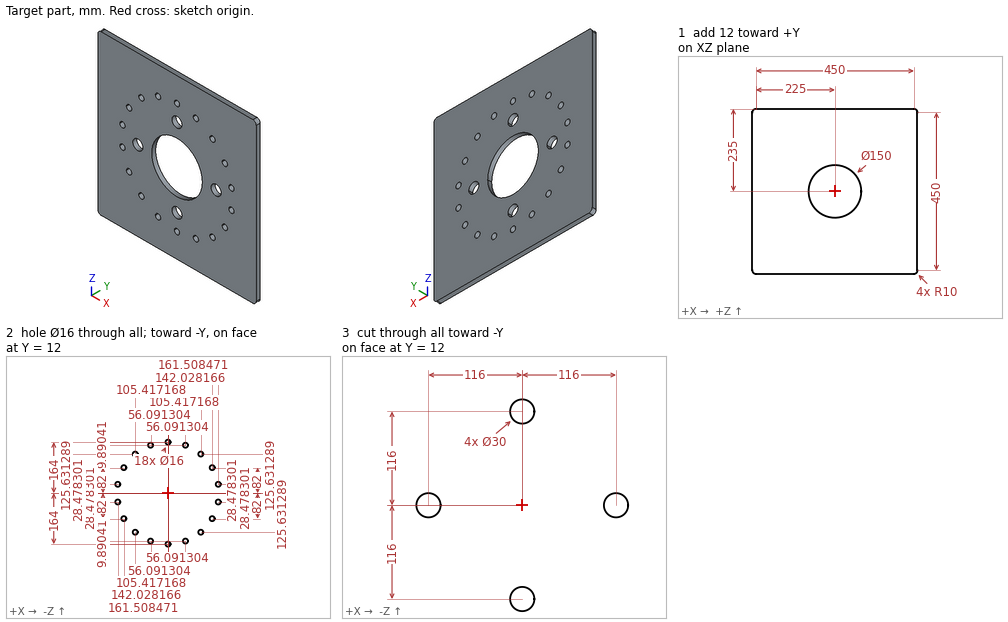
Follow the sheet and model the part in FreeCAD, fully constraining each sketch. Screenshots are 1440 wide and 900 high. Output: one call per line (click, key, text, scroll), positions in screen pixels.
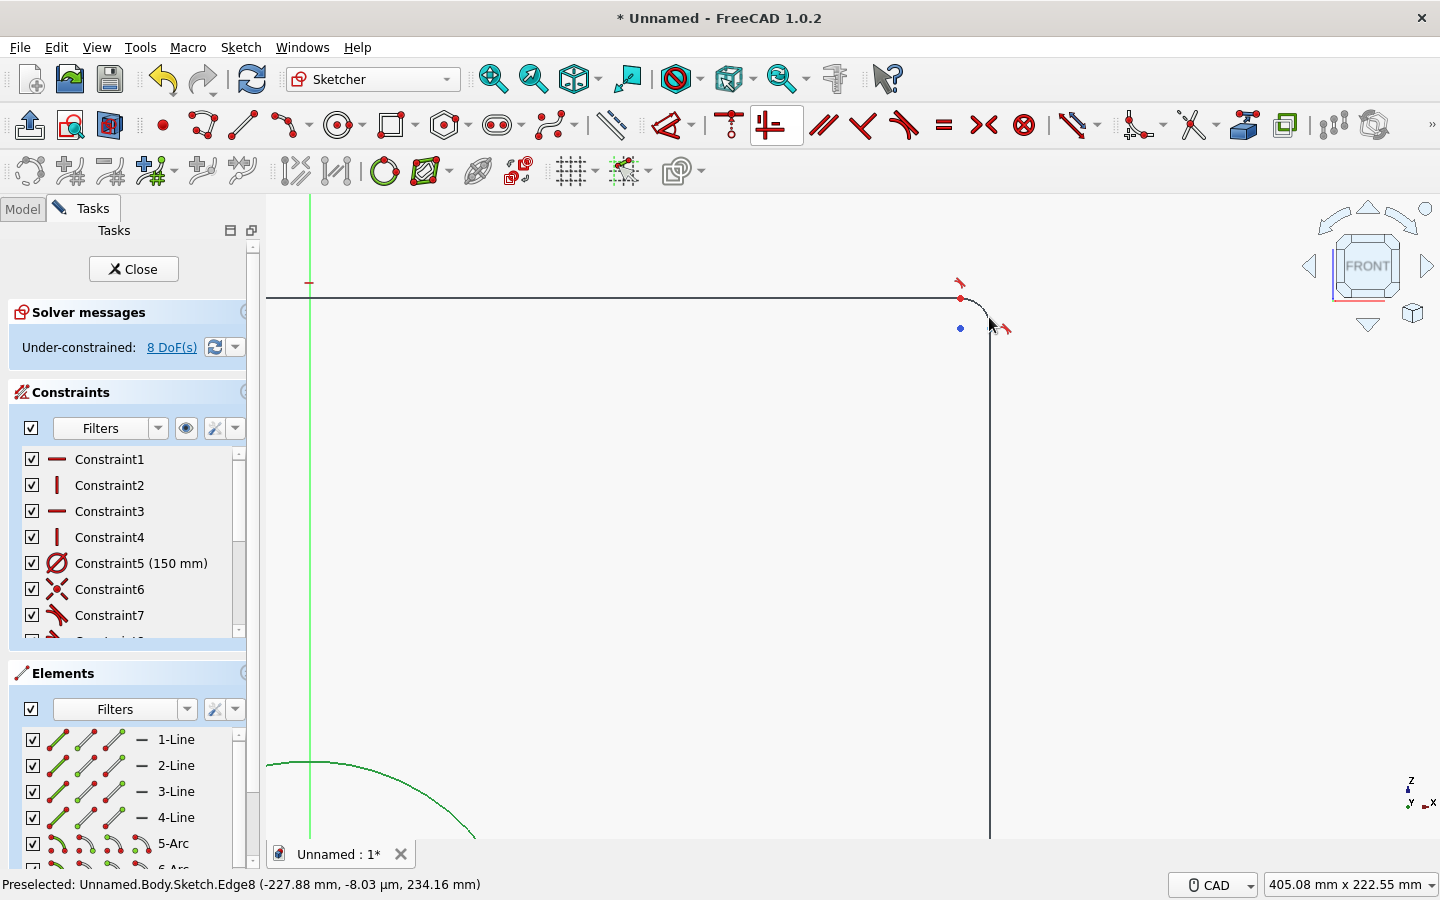
click(987, 315)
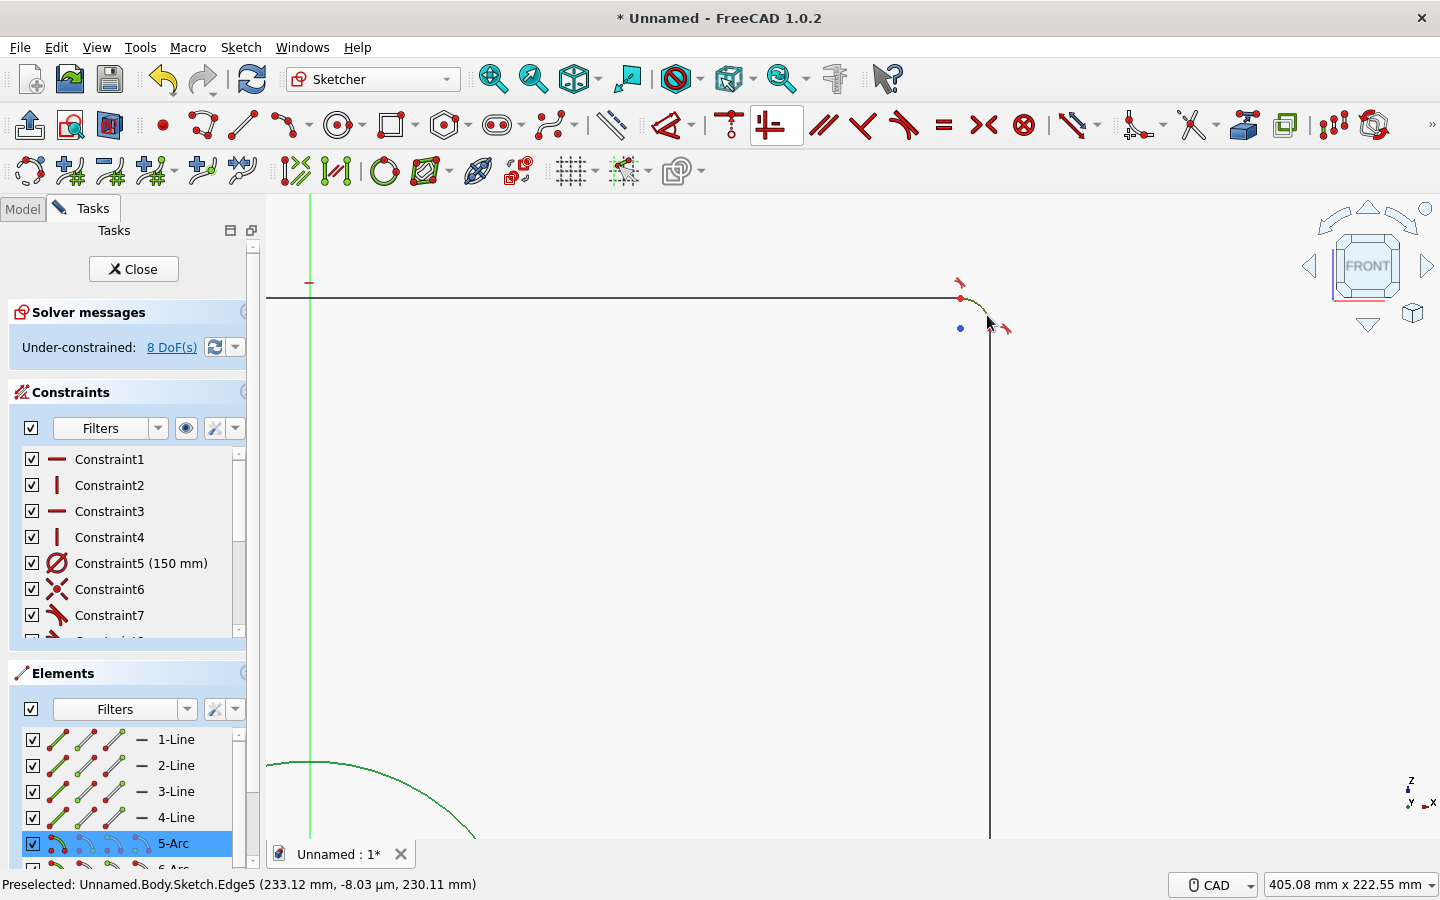
scroll(989, 317, down, 6)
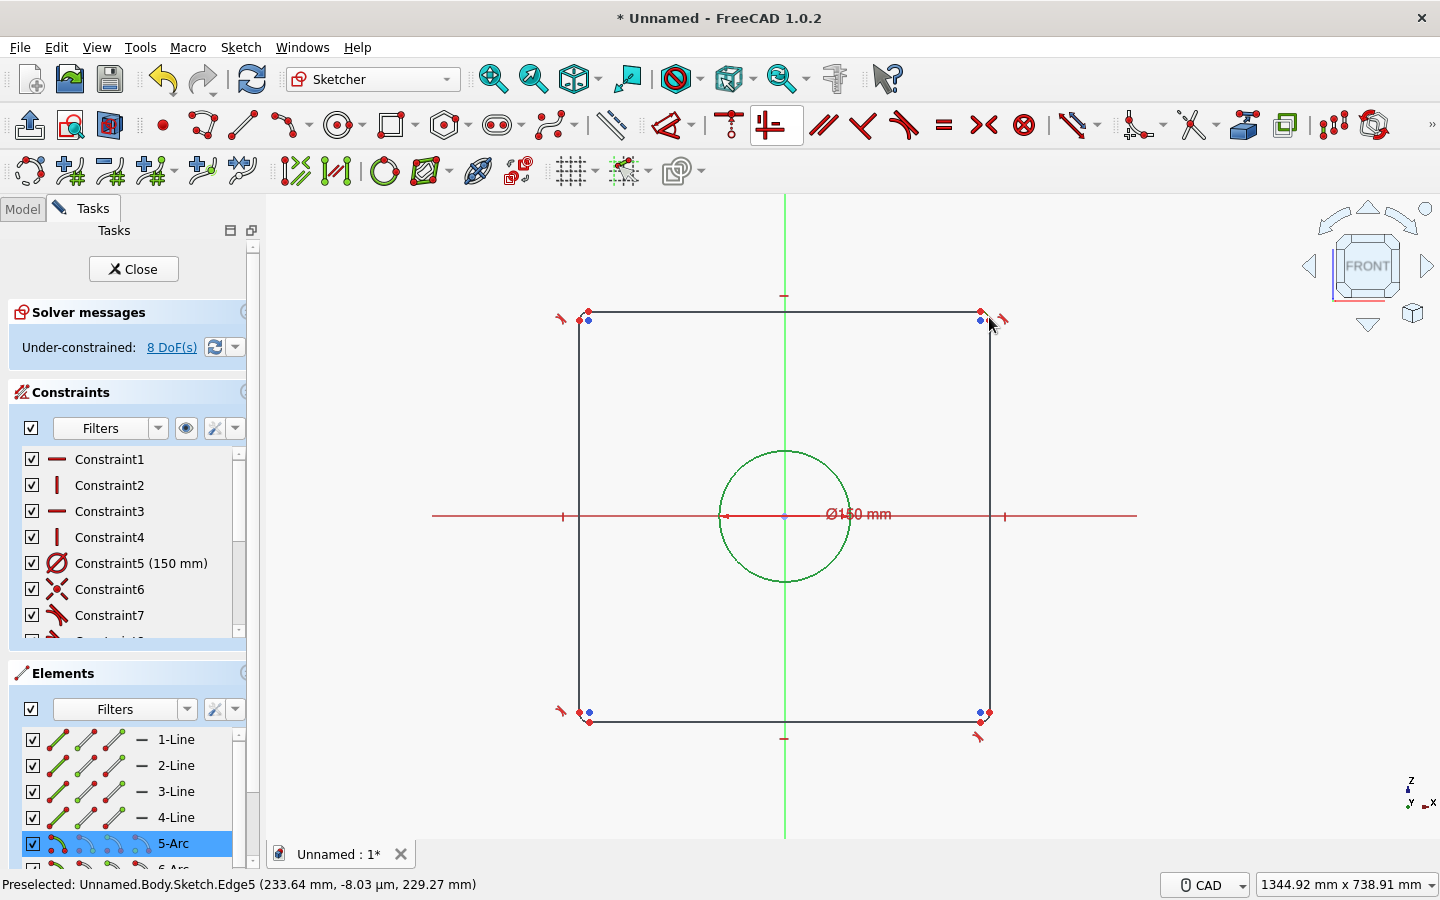
scroll(985, 721, up, 6)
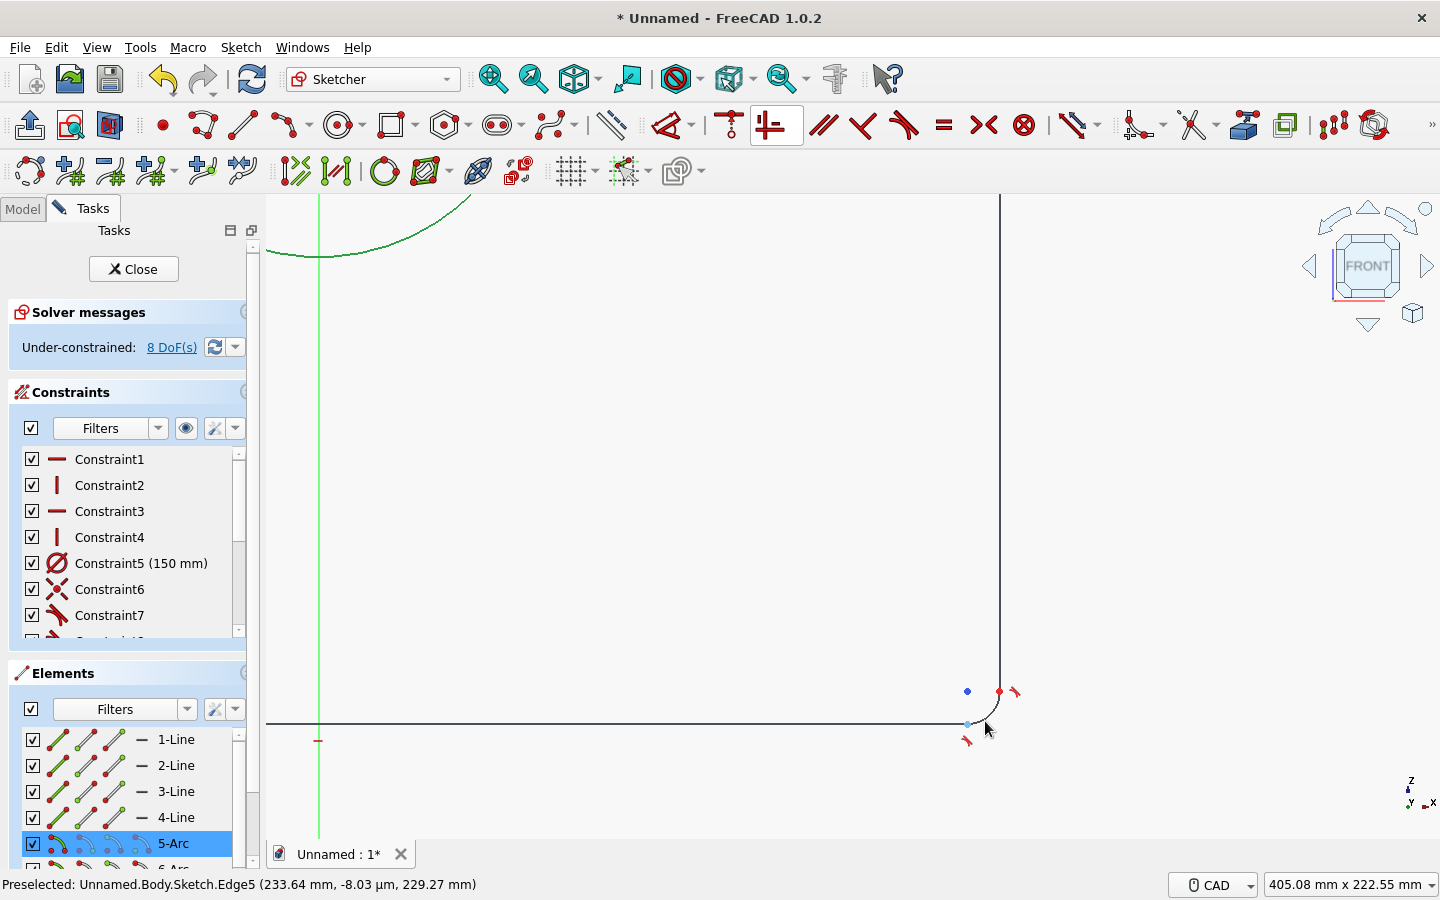
click(982, 721)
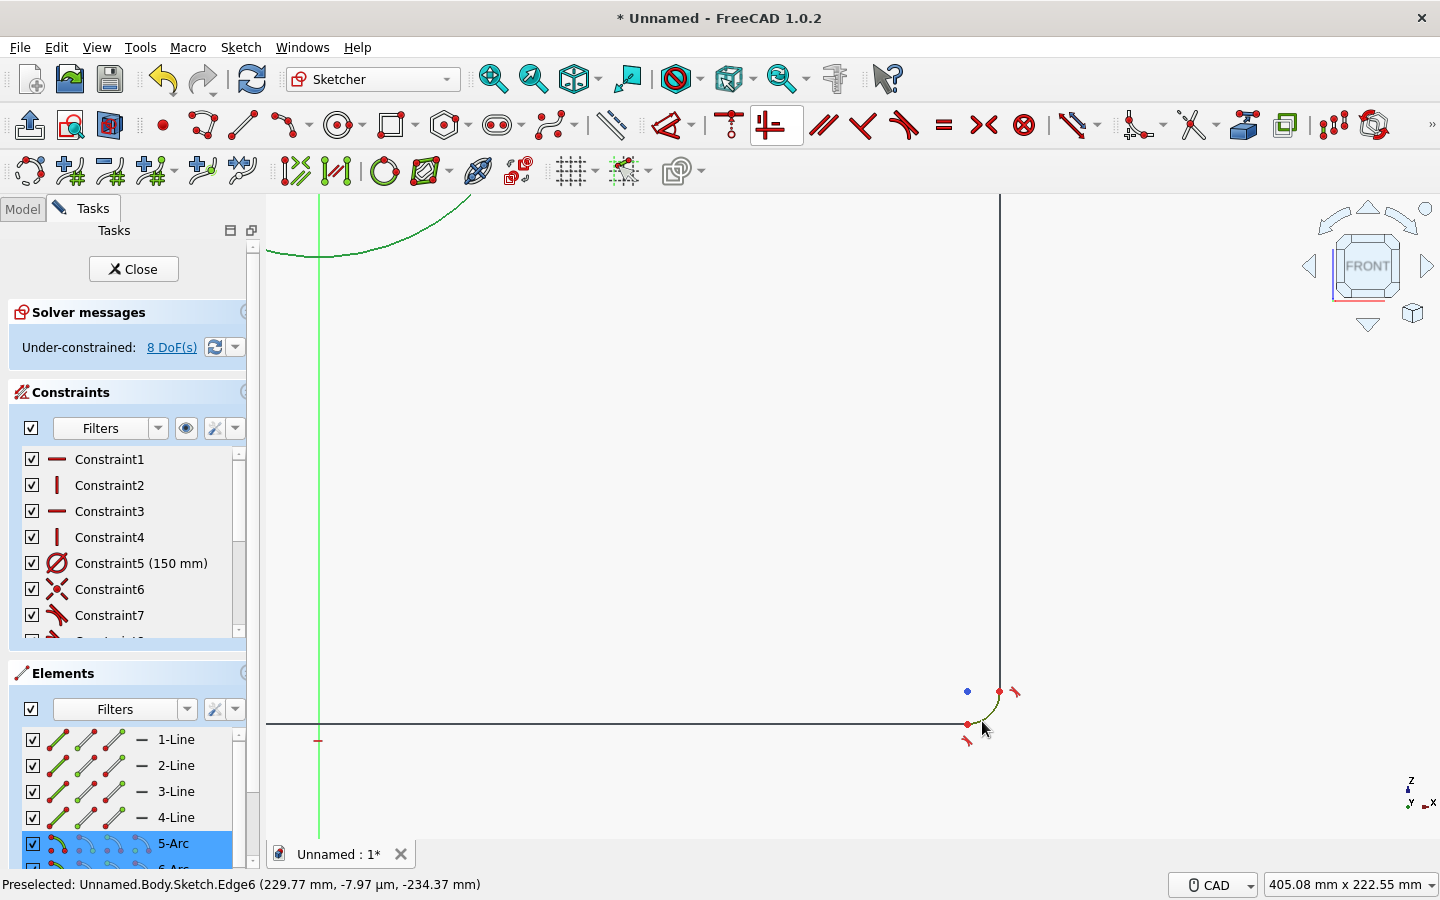
scroll(985, 722, down, 6)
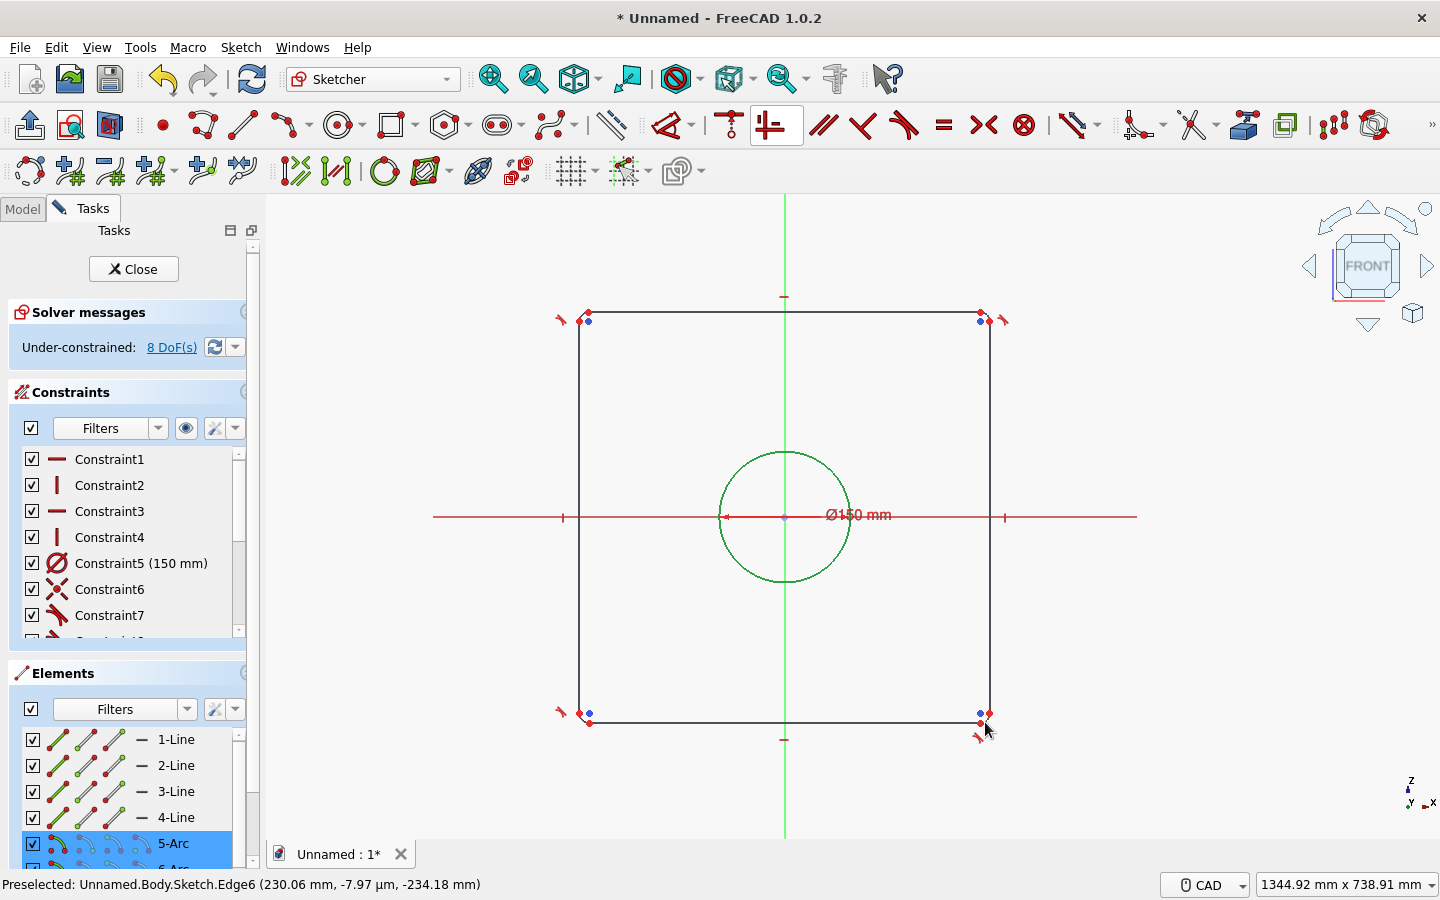
scroll(581, 718, up, 6)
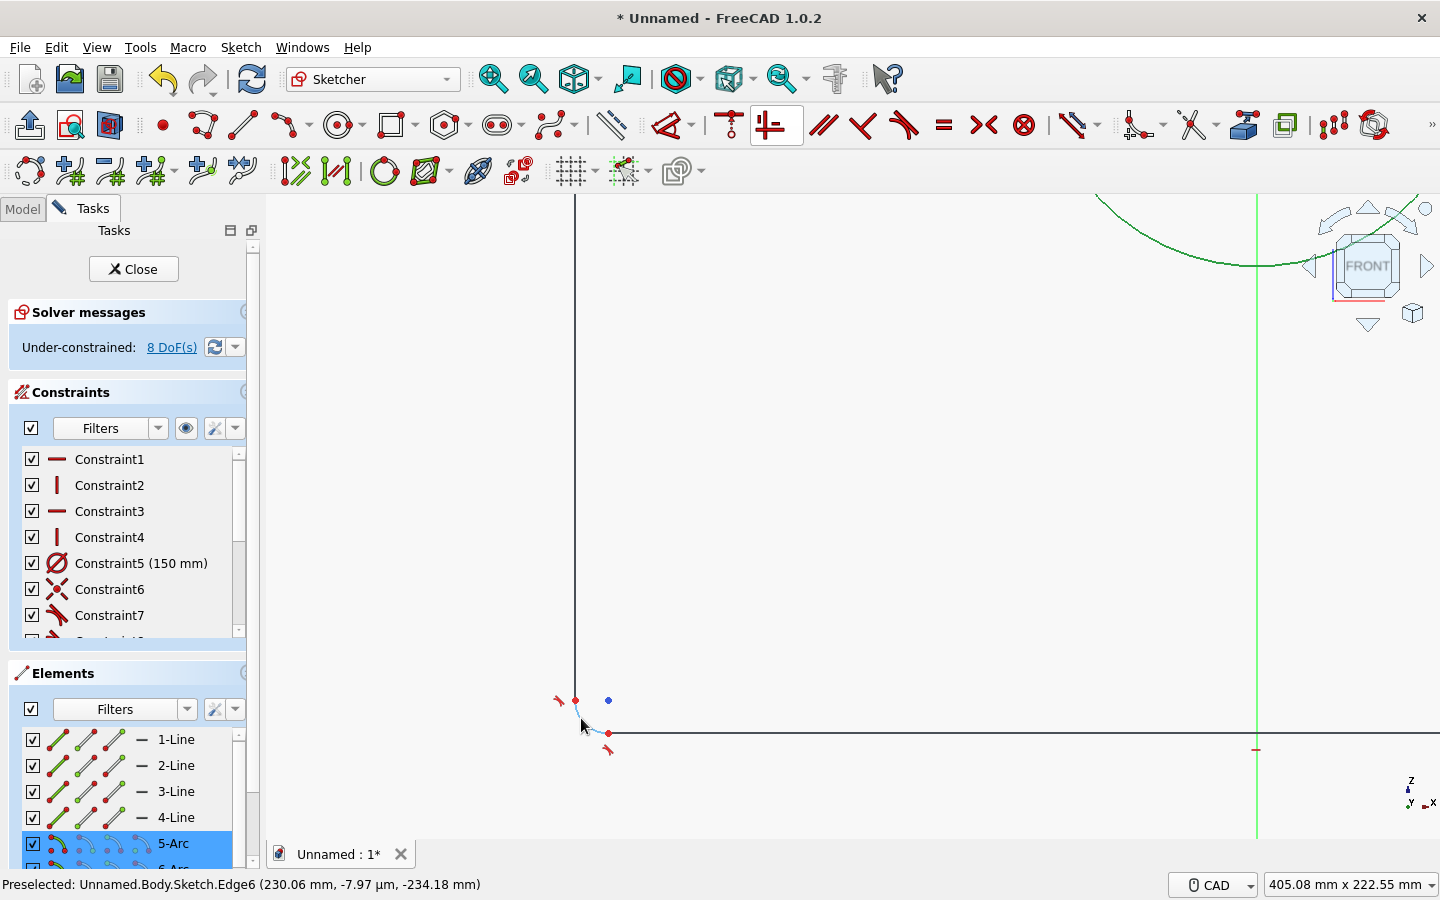
click(579, 715)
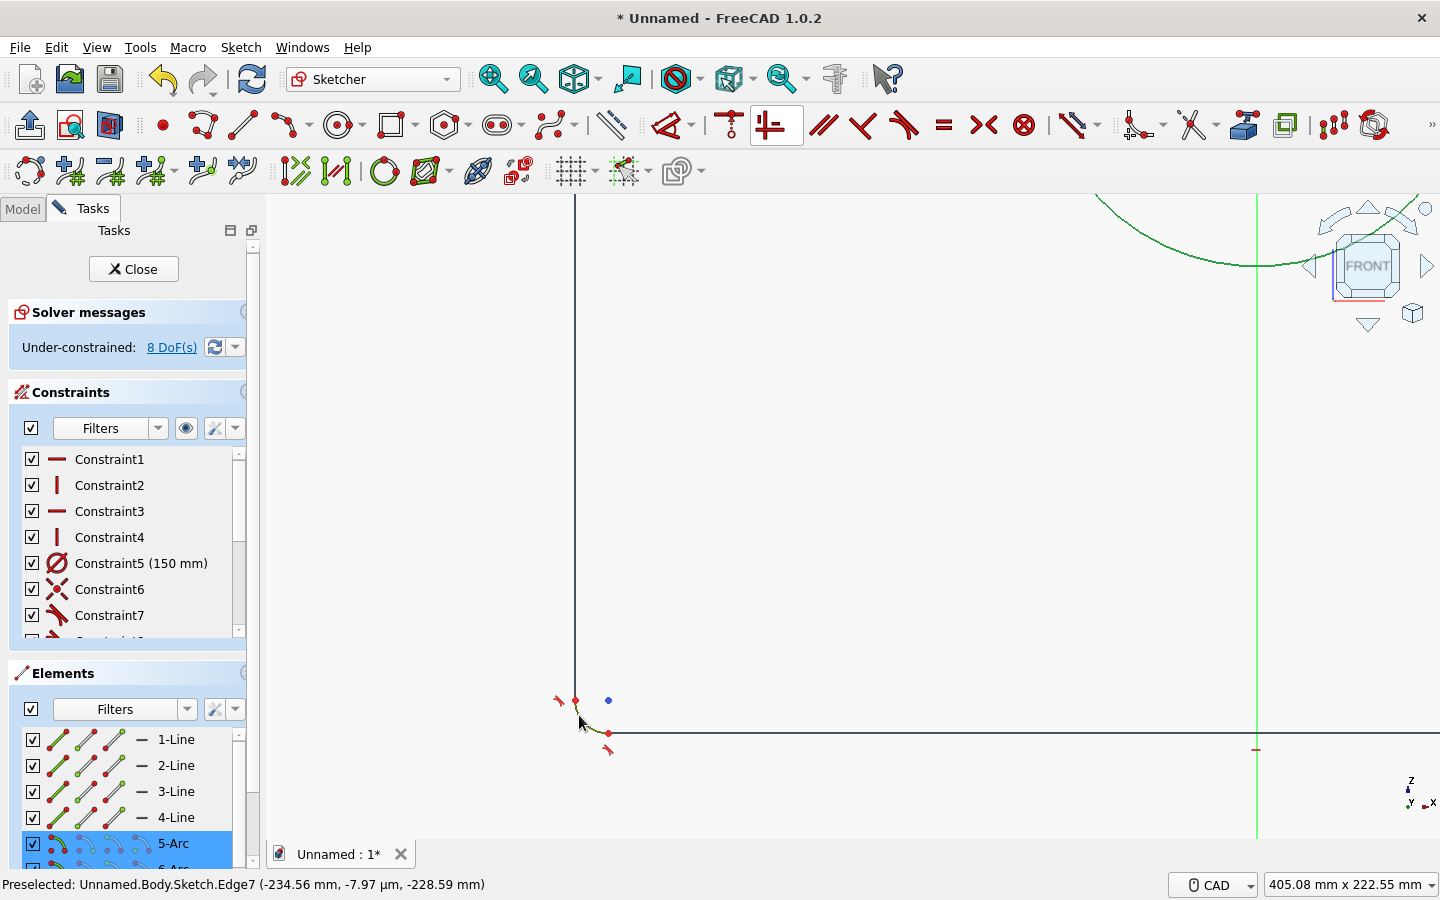
scroll(581, 718, down, 6)